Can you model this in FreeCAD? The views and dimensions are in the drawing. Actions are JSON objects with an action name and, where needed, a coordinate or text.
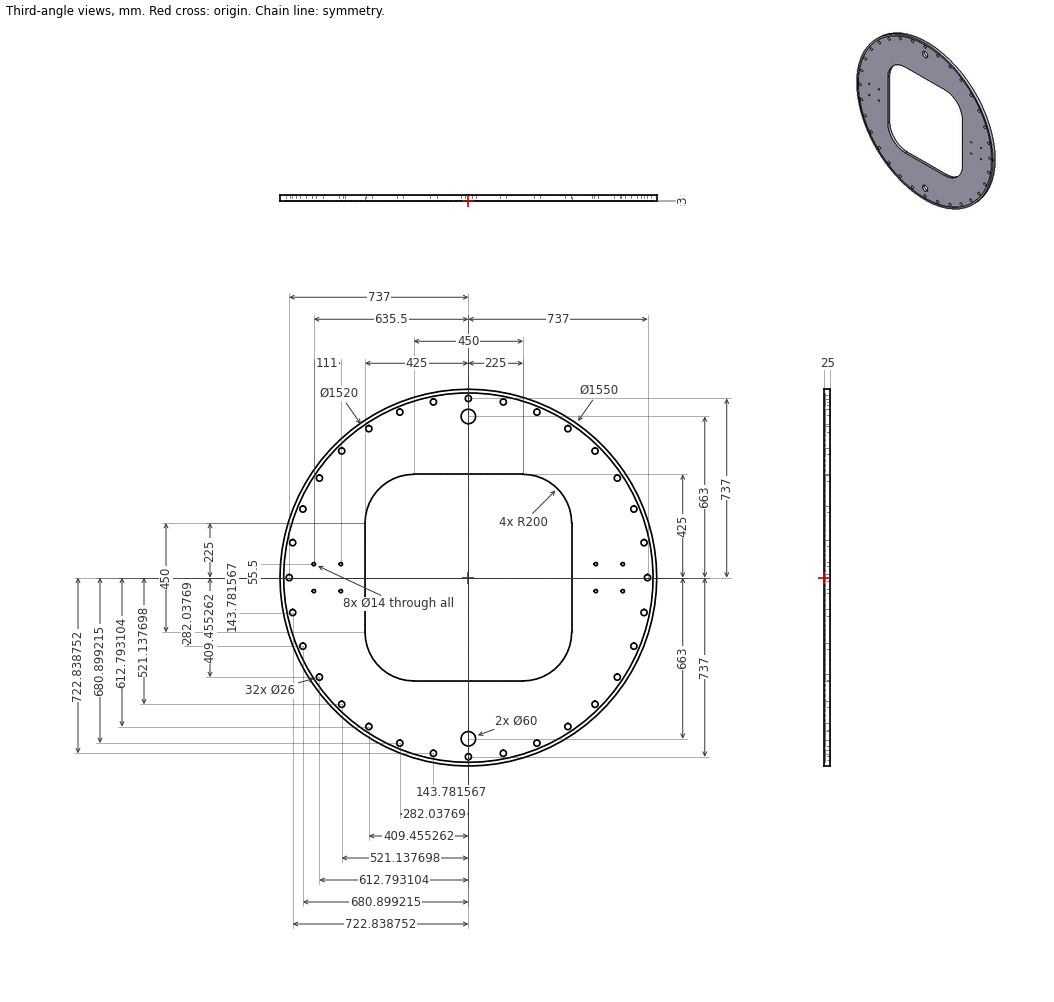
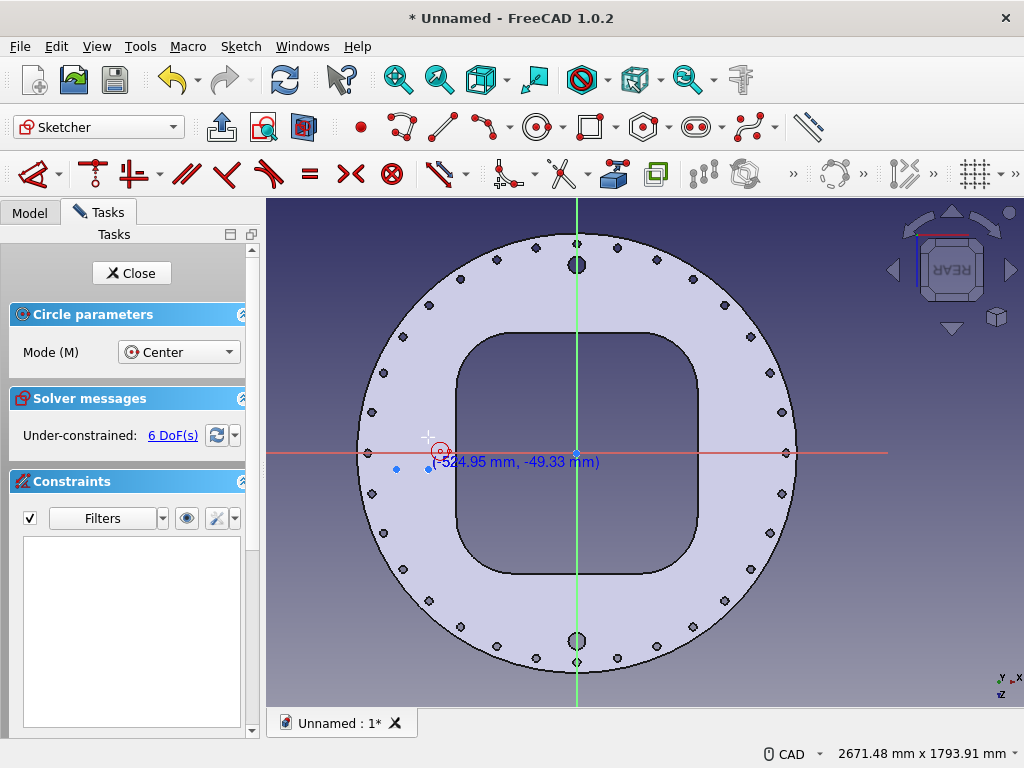
{"action": "left_click", "coordinate": [428, 437]}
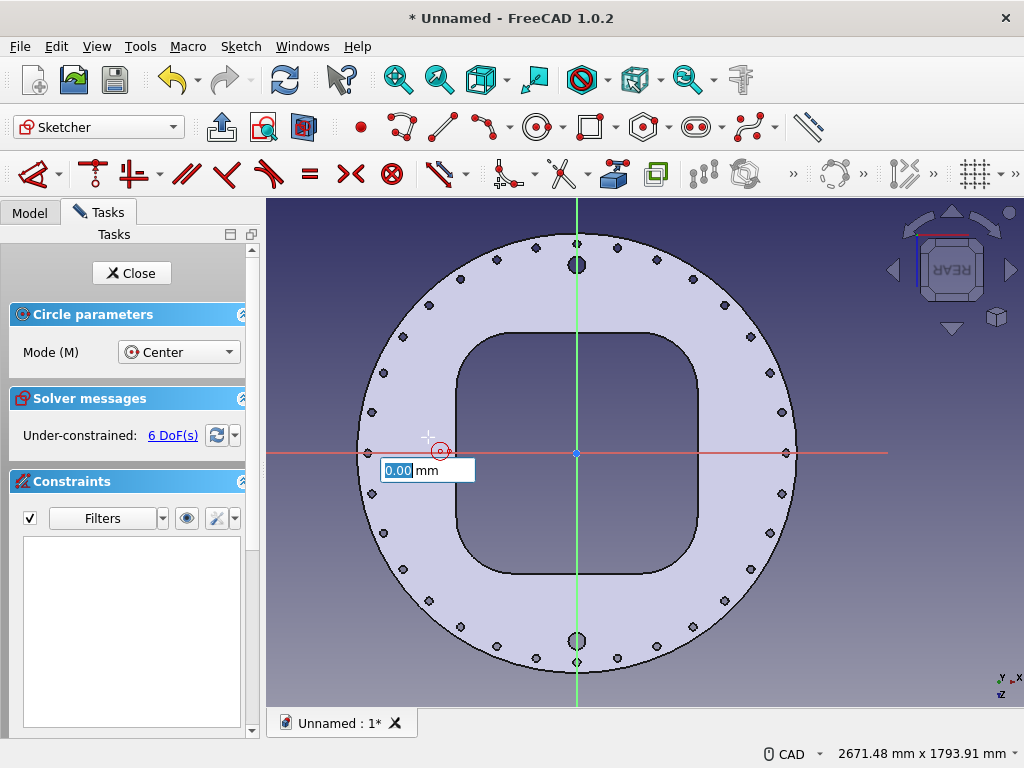
{"action": "scroll", "coordinate": [430, 436], "scroll_direction": "up", "scroll_amount": 11}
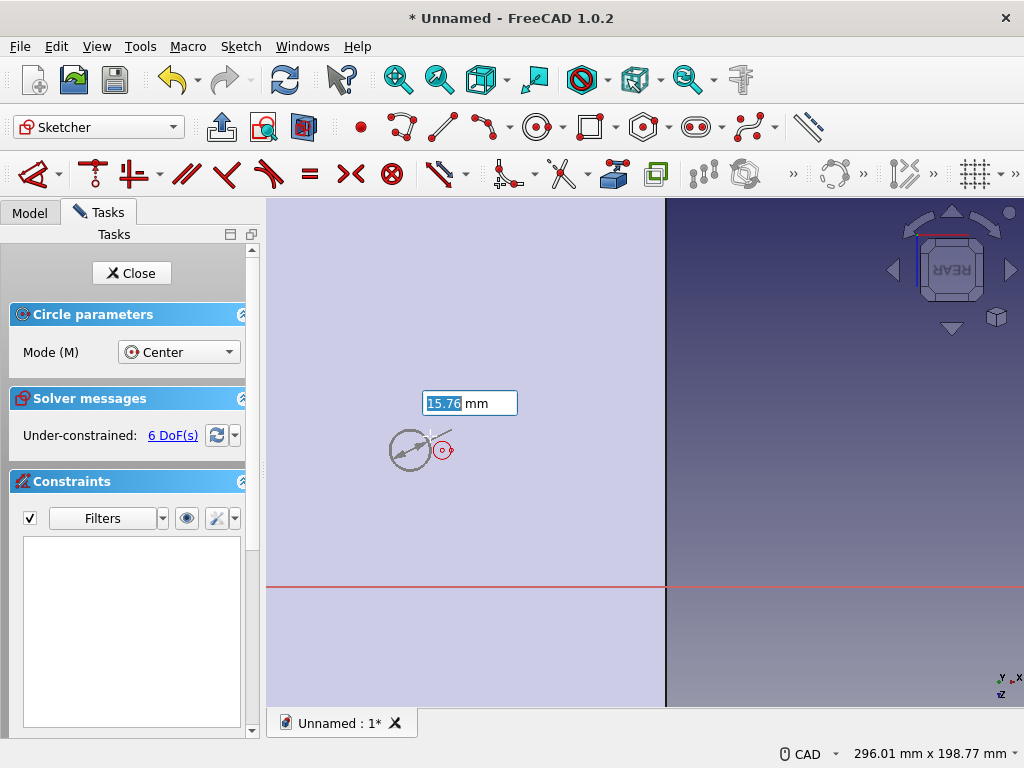
{"action": "left_click", "coordinate": [424, 432]}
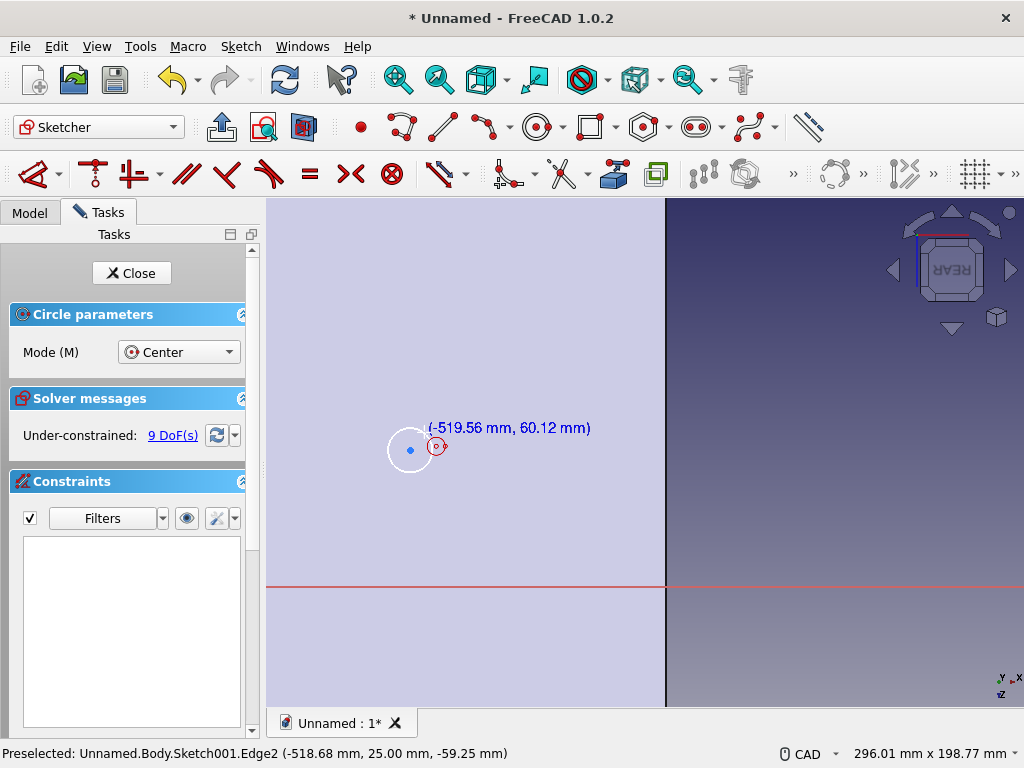
{"action": "scroll", "coordinate": [430, 436], "scroll_direction": "down", "scroll_amount": 11}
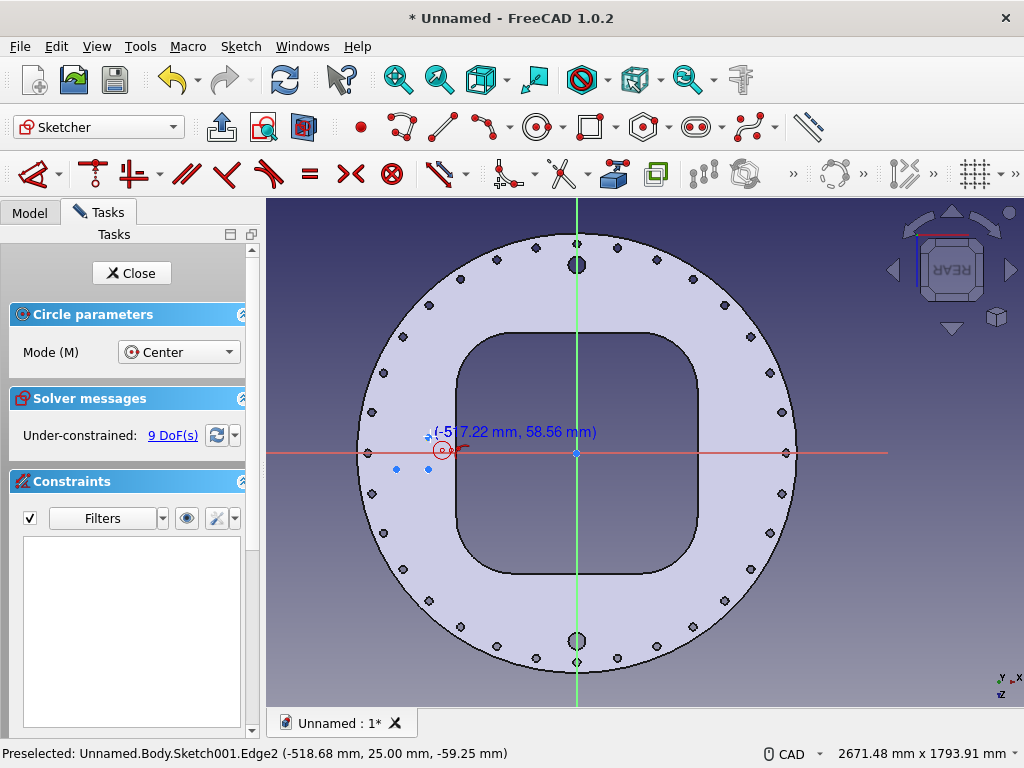
{"action": "scroll", "coordinate": [397, 437], "scroll_direction": "up", "scroll_amount": 13}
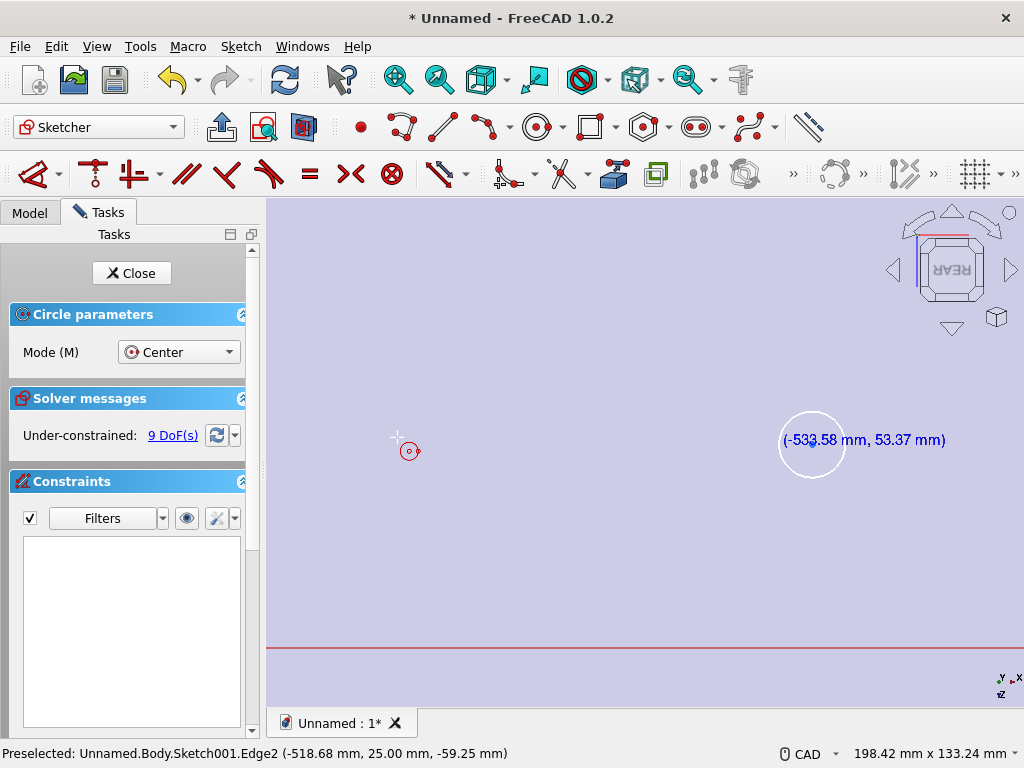
{"action": "scroll", "coordinate": [397, 437], "scroll_direction": "down", "scroll_amount": 13}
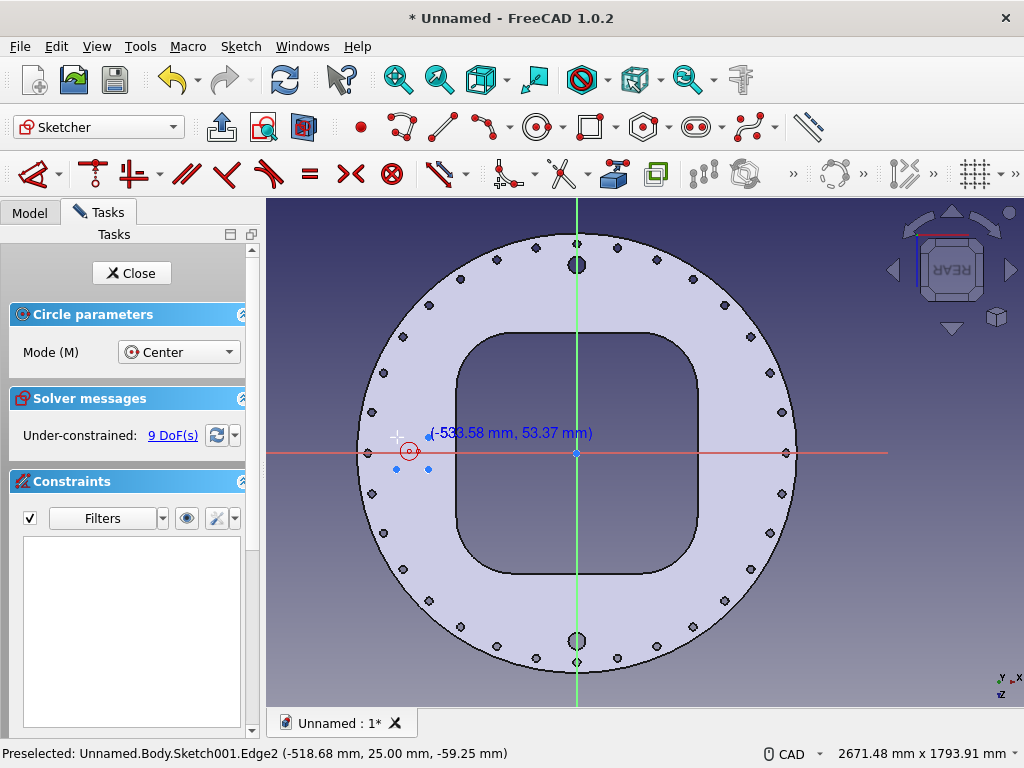
{"action": "left_click", "coordinate": [397, 437]}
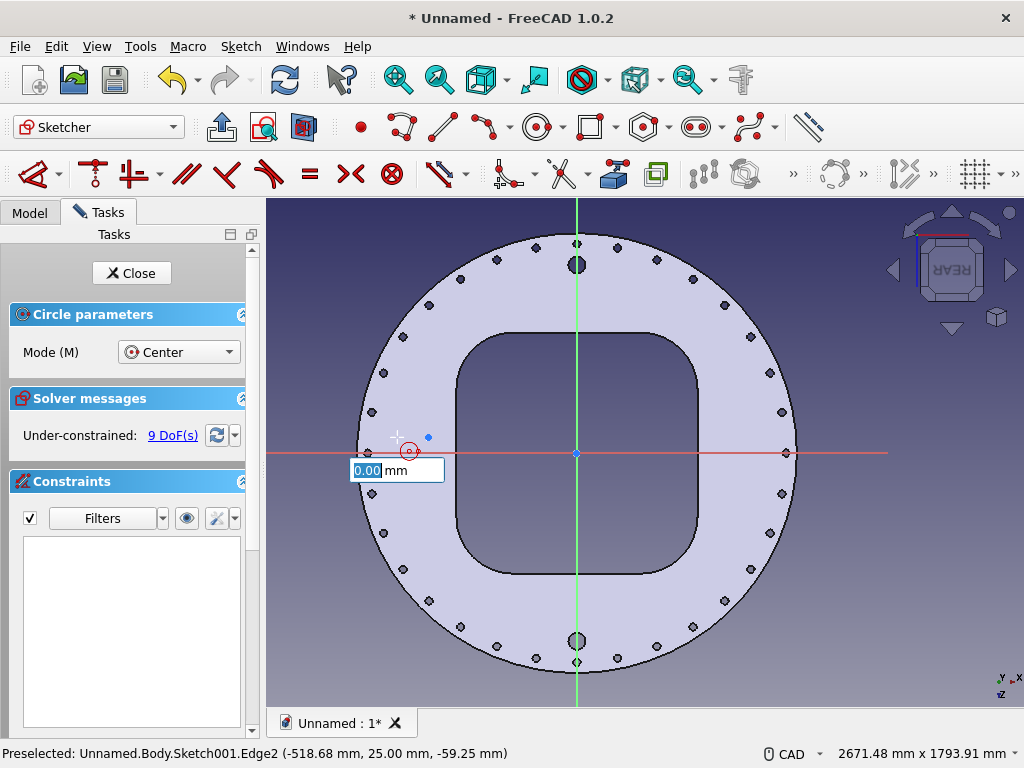
{"action": "scroll", "coordinate": [398, 436], "scroll_direction": "up", "scroll_amount": 11}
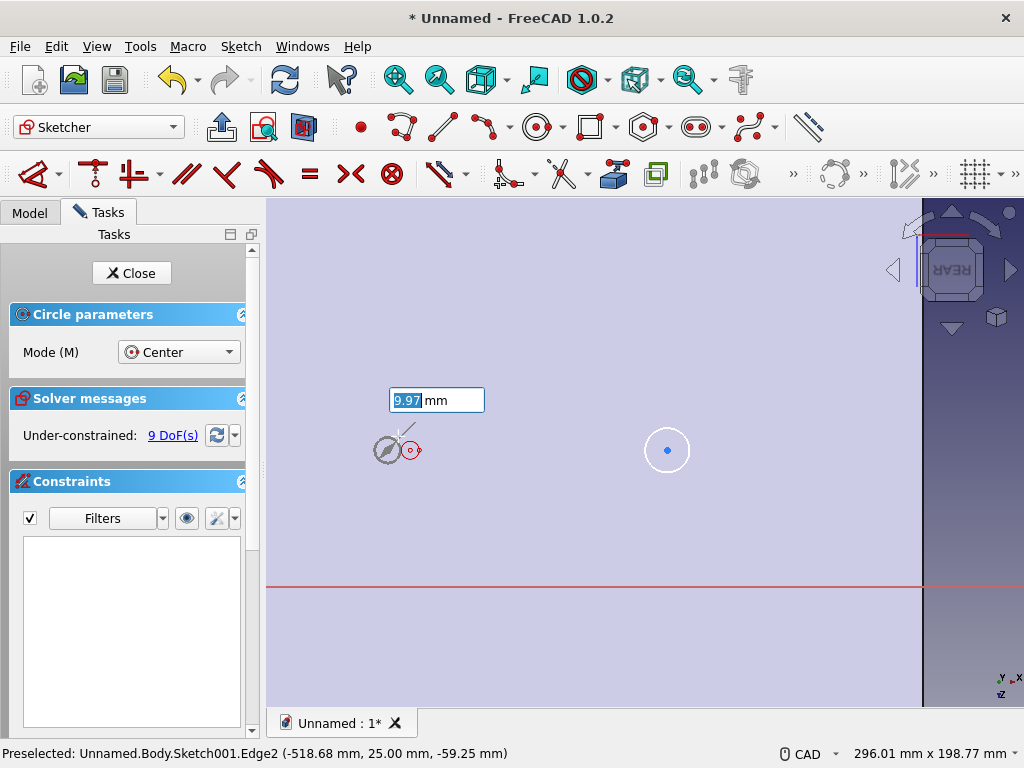
{"action": "left_click", "coordinate": [397, 432]}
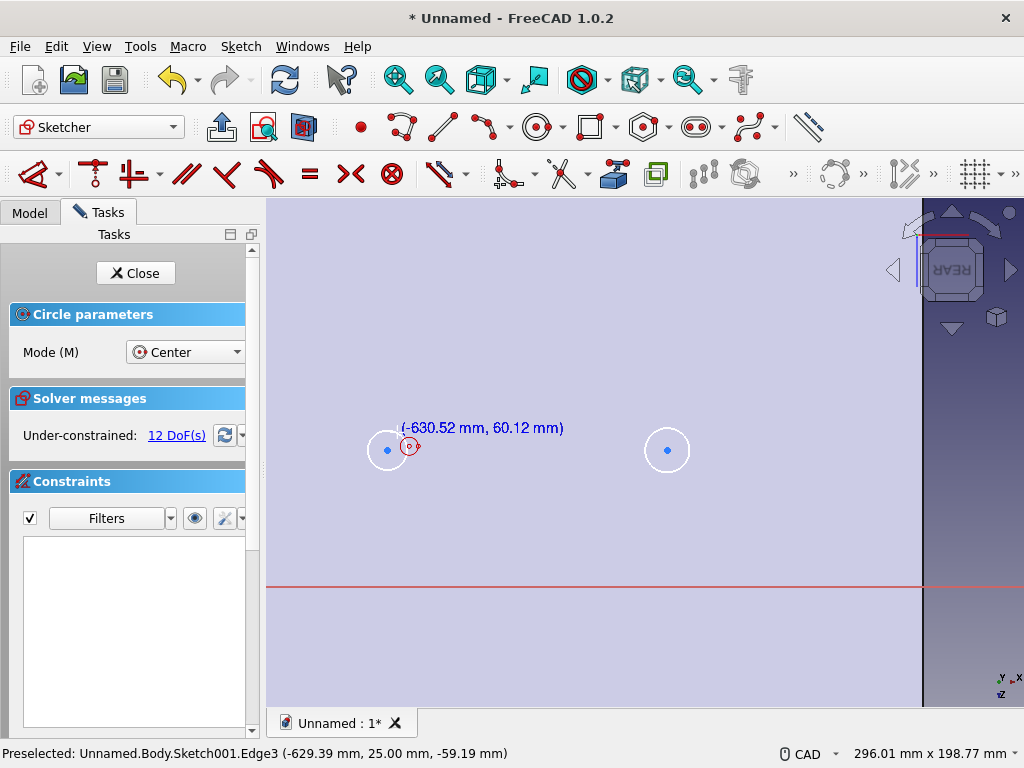
{"action": "scroll", "coordinate": [398, 436], "scroll_direction": "down", "scroll_amount": 11}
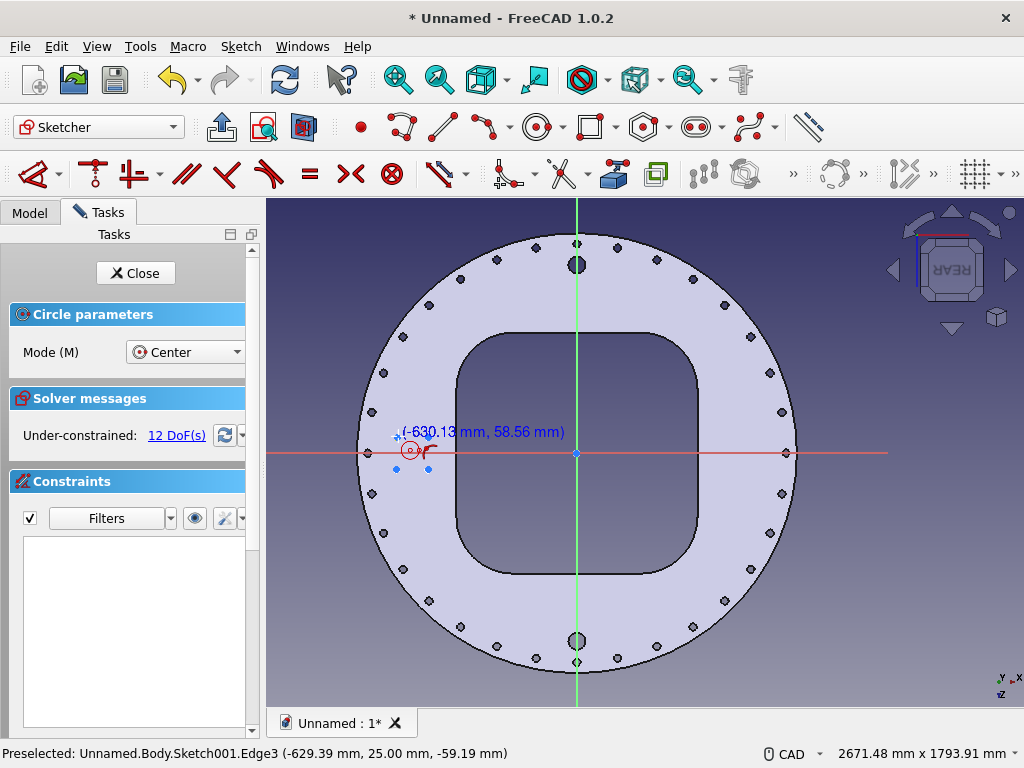
{"action": "scroll", "coordinate": [757, 437], "scroll_direction": "up", "scroll_amount": 13}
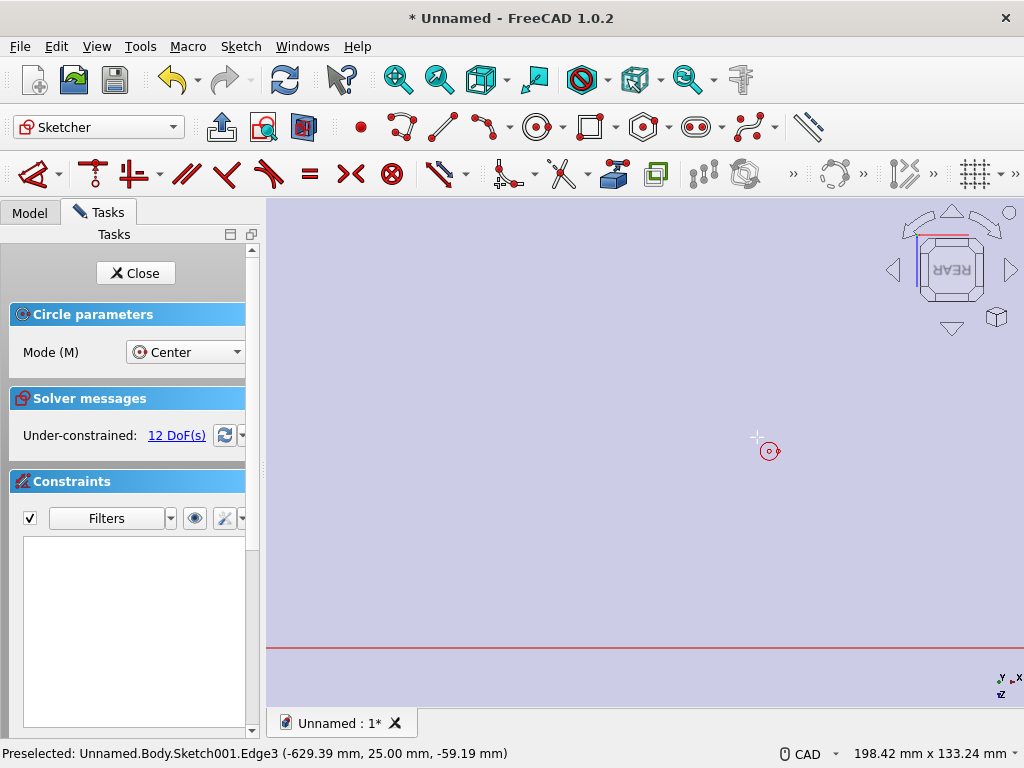
{"action": "scroll", "coordinate": [757, 437], "scroll_direction": "down", "scroll_amount": 13}